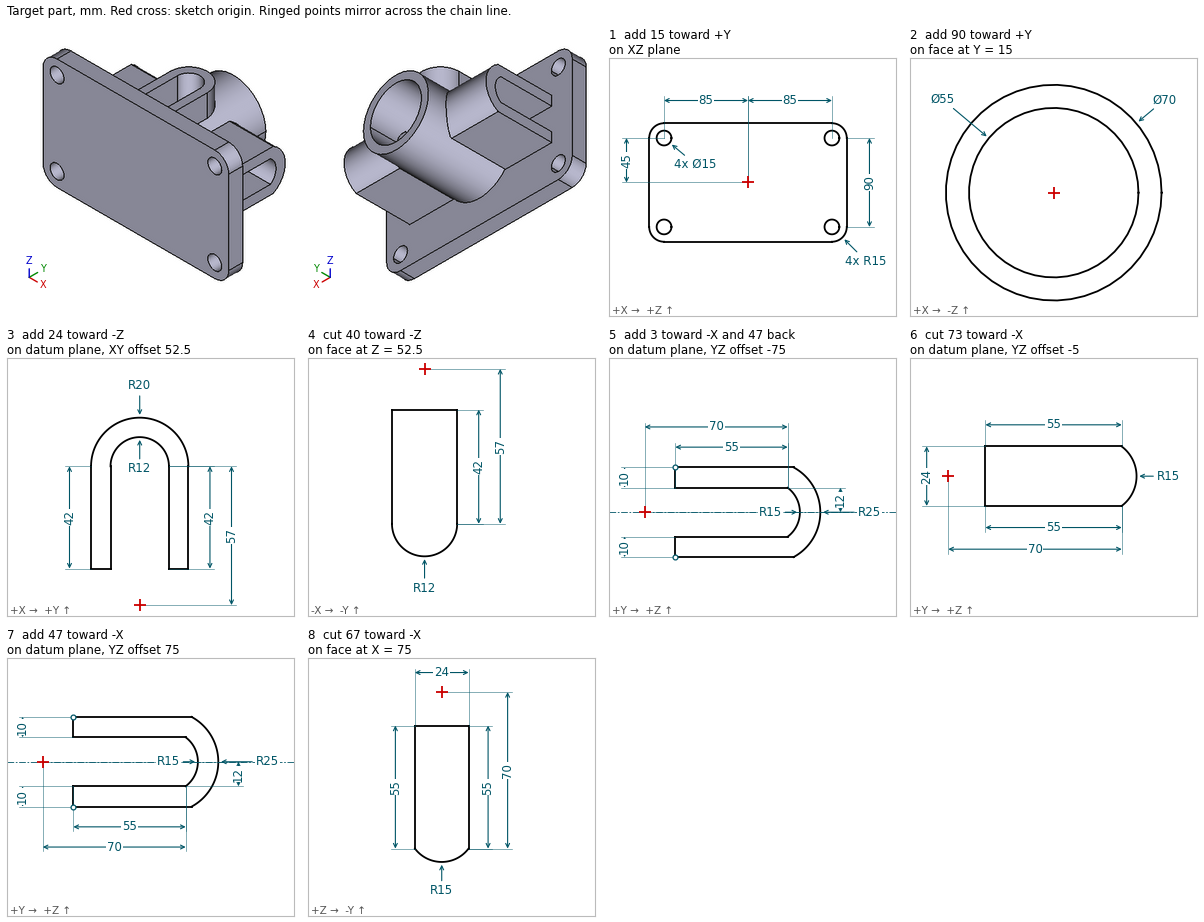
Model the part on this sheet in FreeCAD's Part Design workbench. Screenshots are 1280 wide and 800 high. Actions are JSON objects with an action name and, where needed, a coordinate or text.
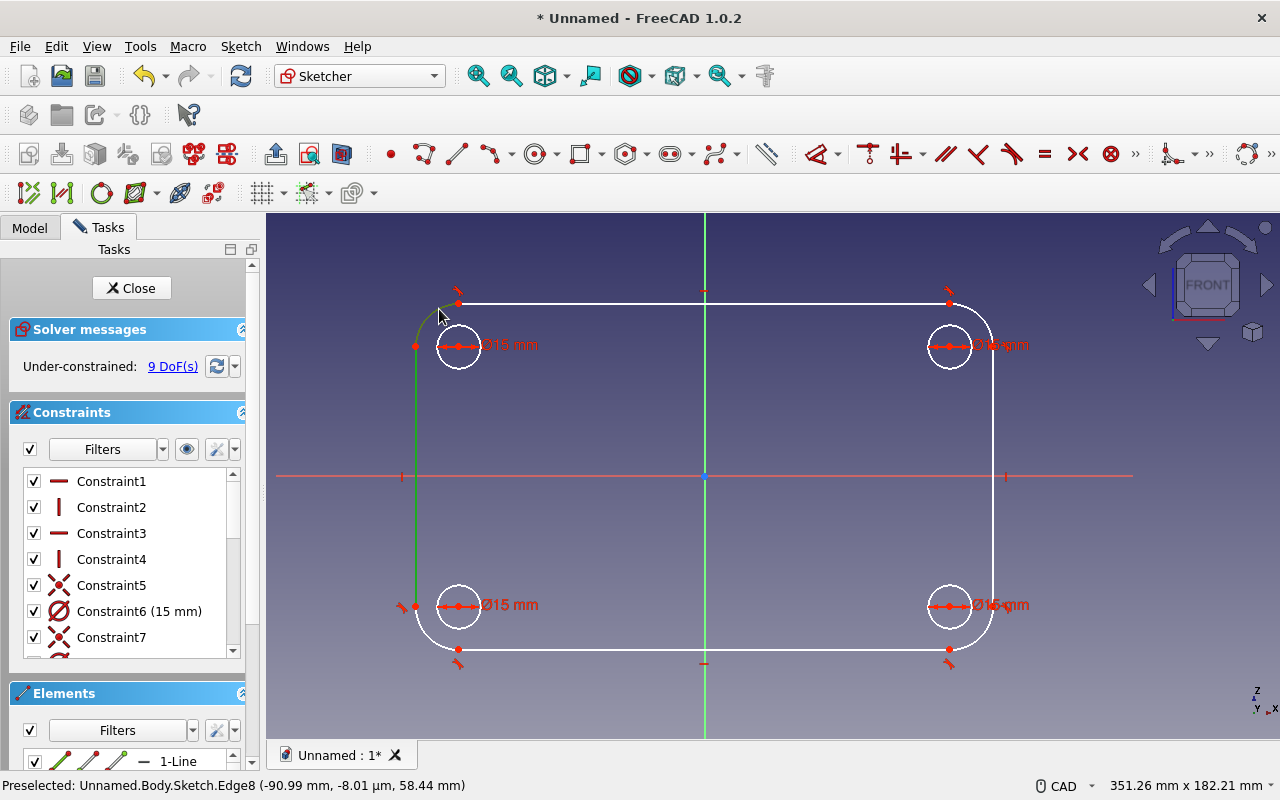
{"action": "key", "text": "t"}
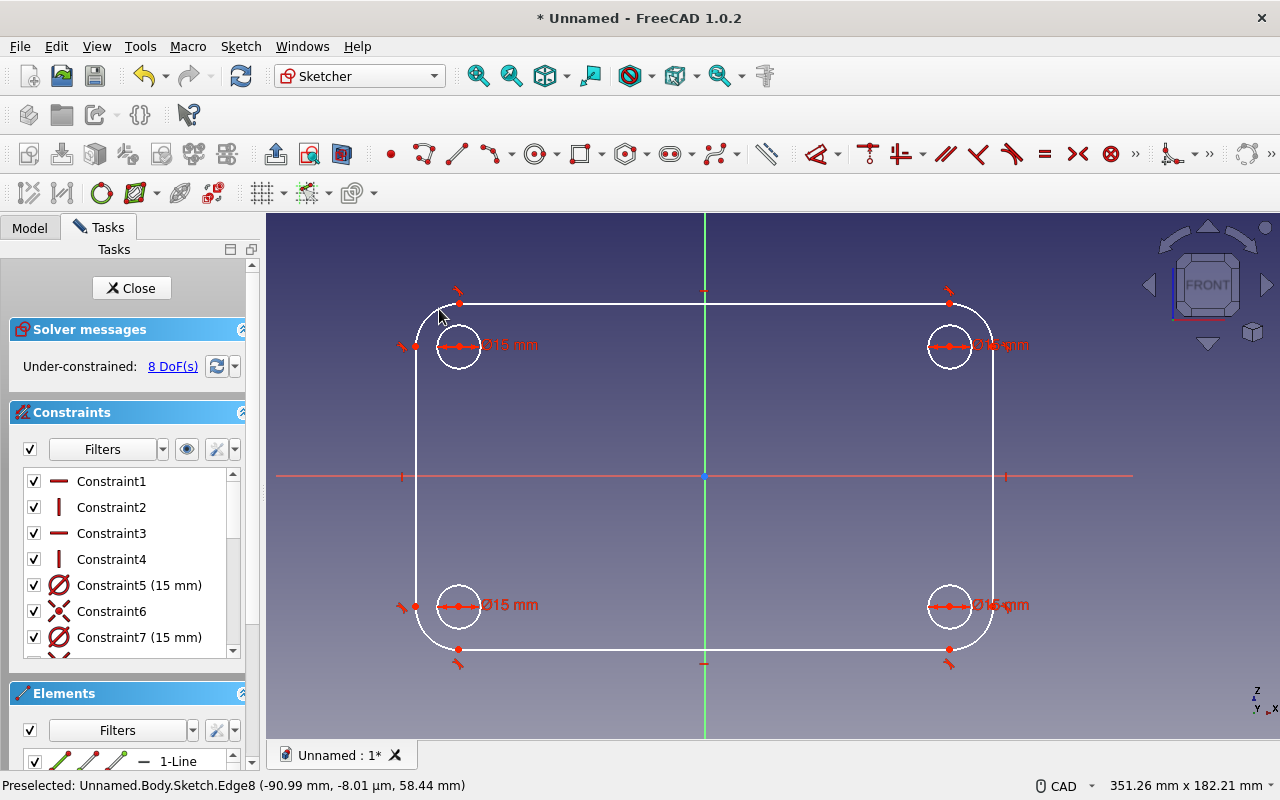
{"action": "left_click", "coordinate": [988, 327]}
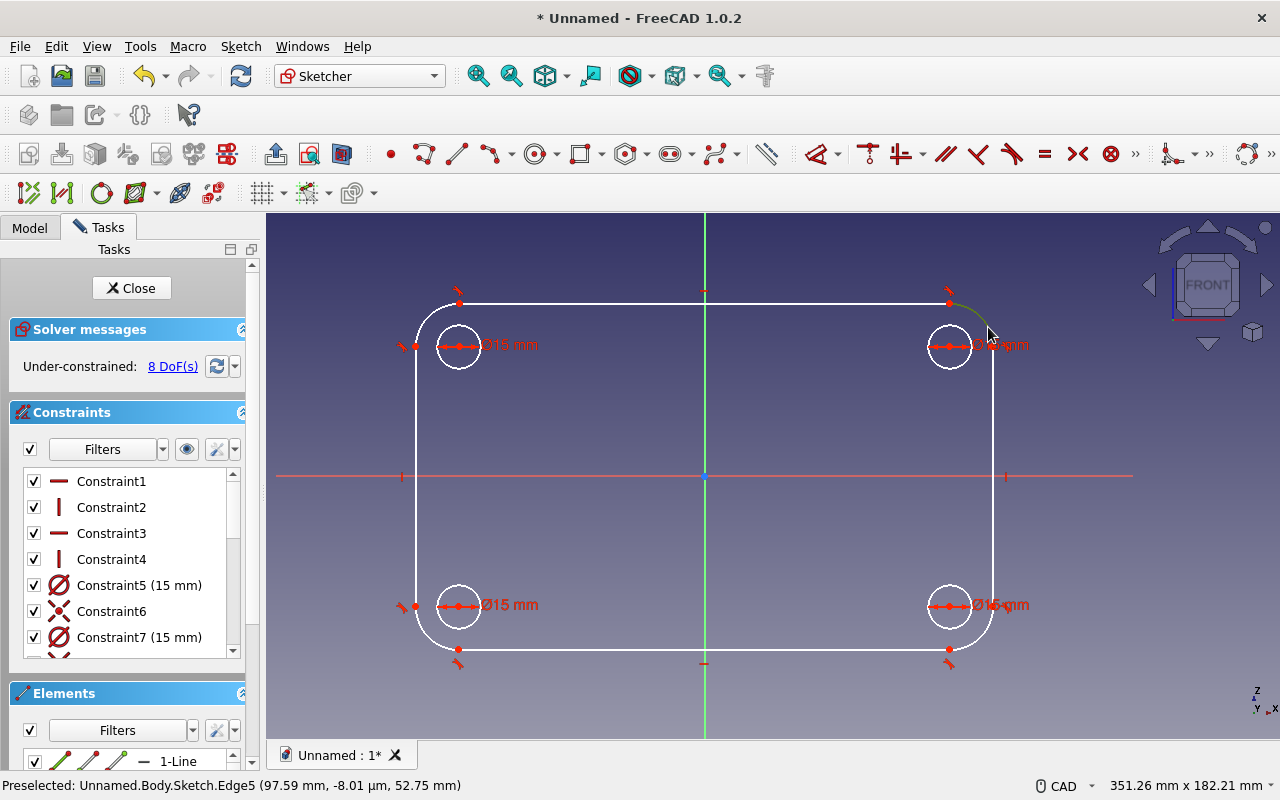
{"action": "left_click", "coordinate": [970, 645]}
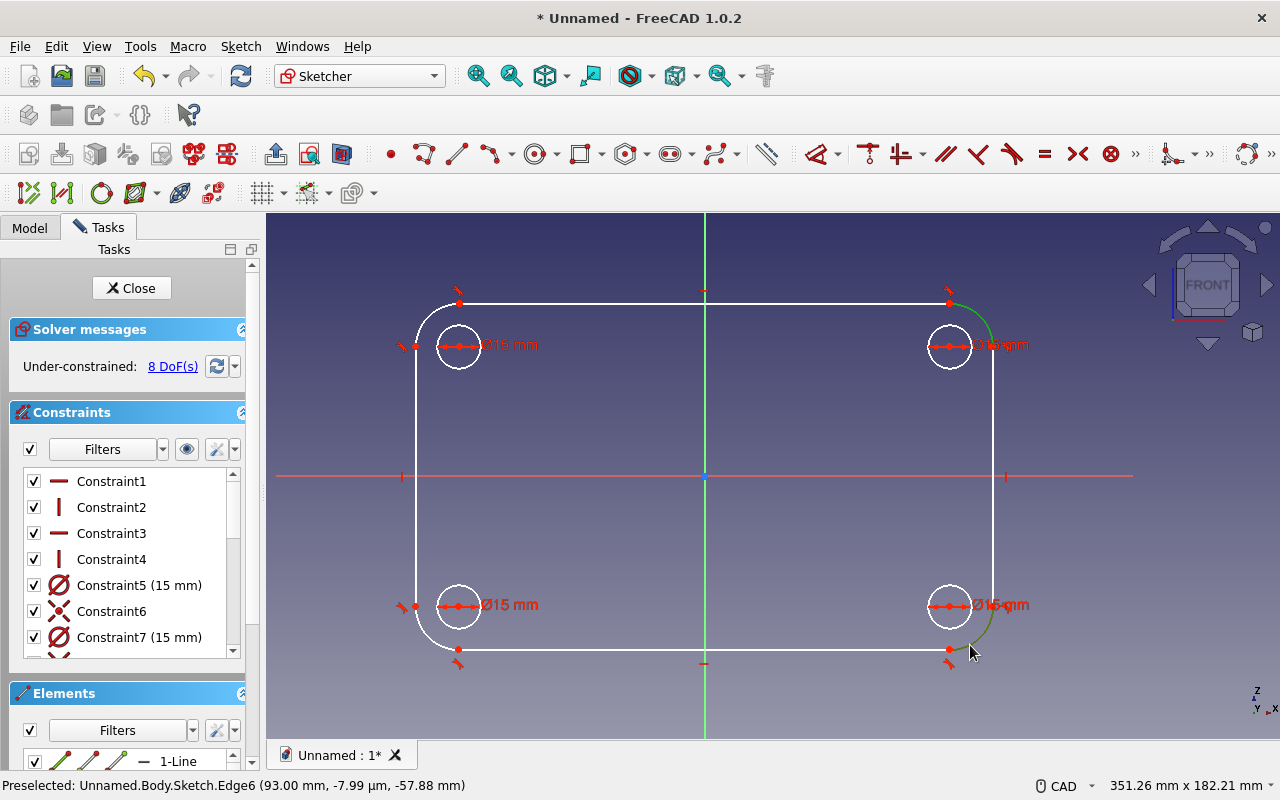
{"action": "left_click", "coordinate": [421, 627]}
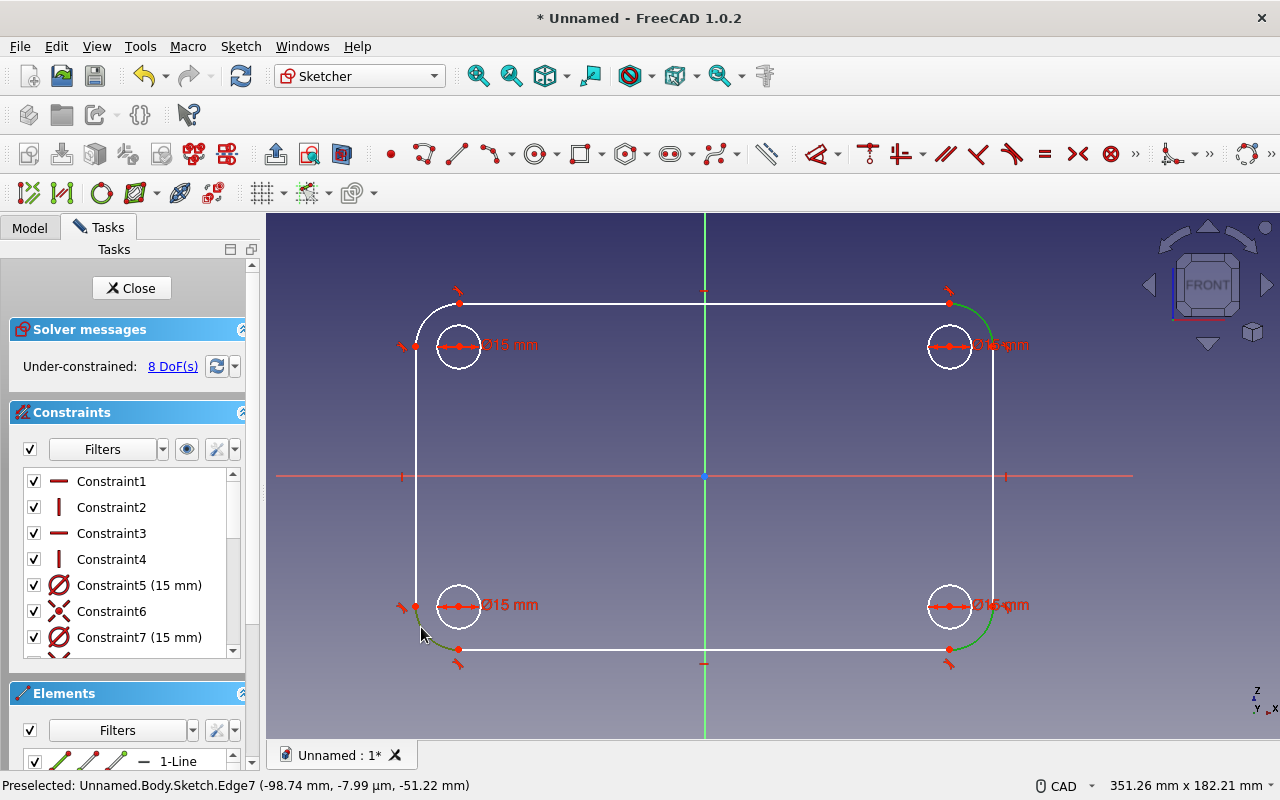
{"action": "left_click", "coordinate": [439, 309]}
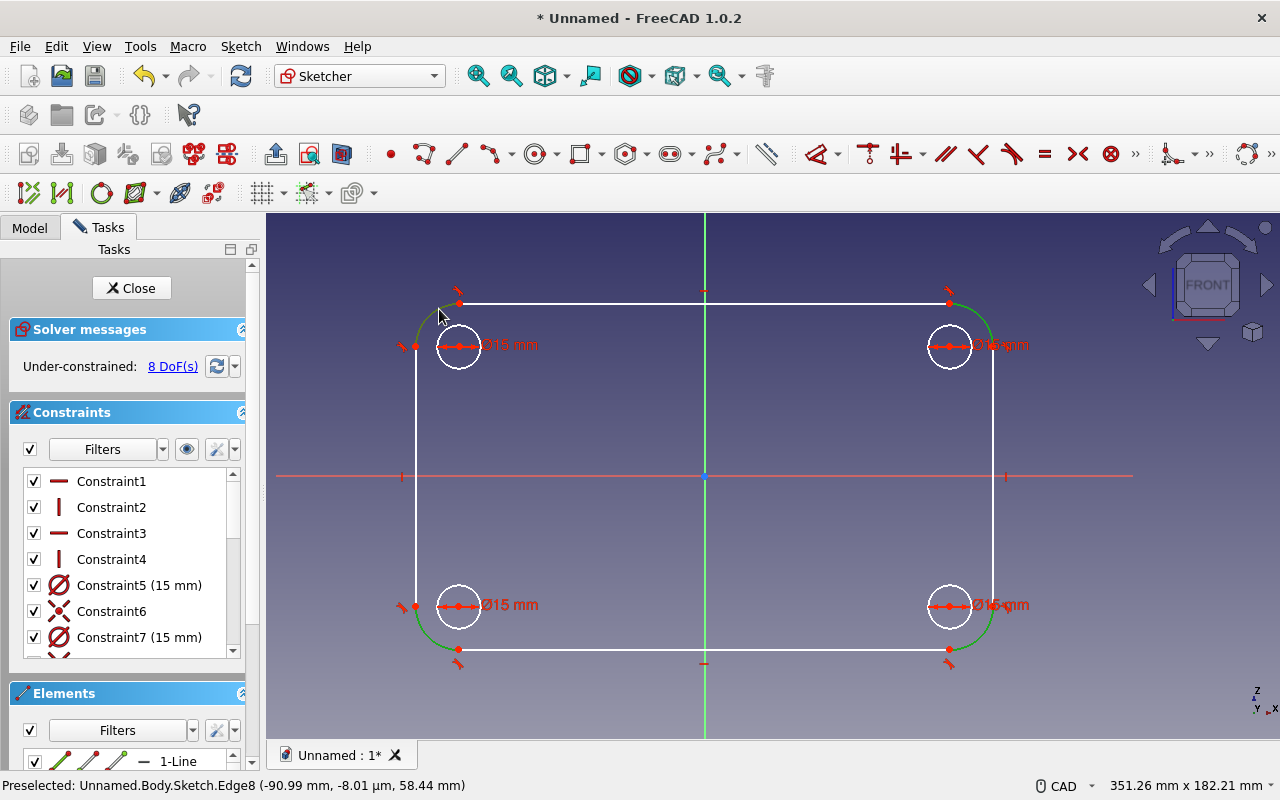
{"action": "key", "text": "e"}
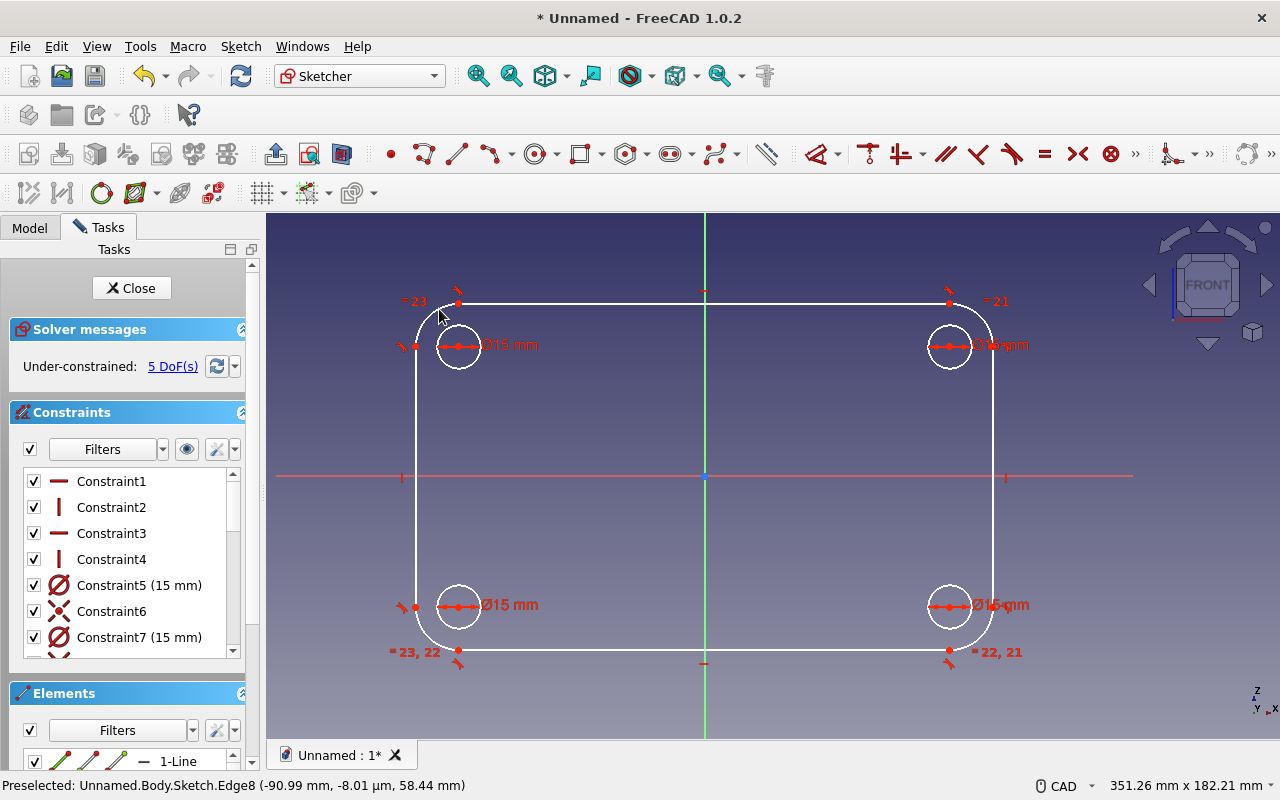
{"action": "left_click", "coordinate": [988, 327]}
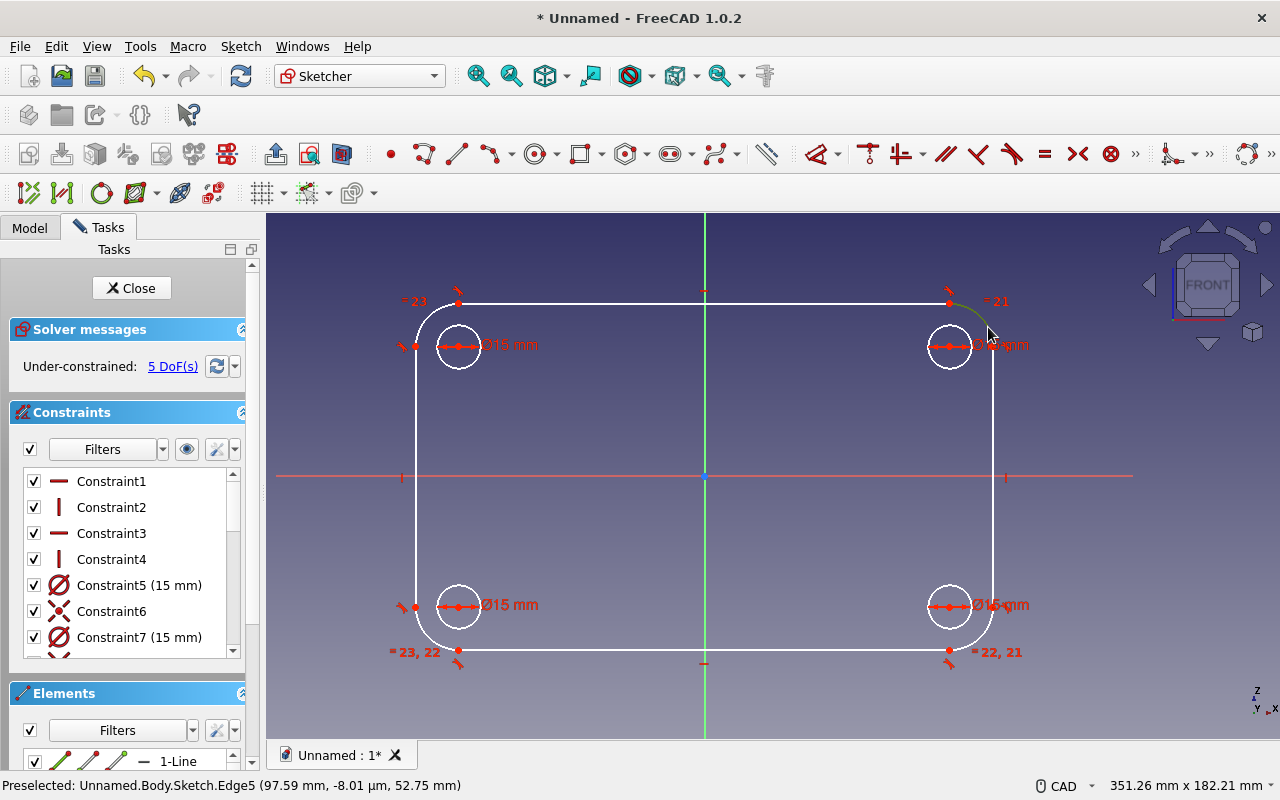
{"action": "key", "text": "k r"}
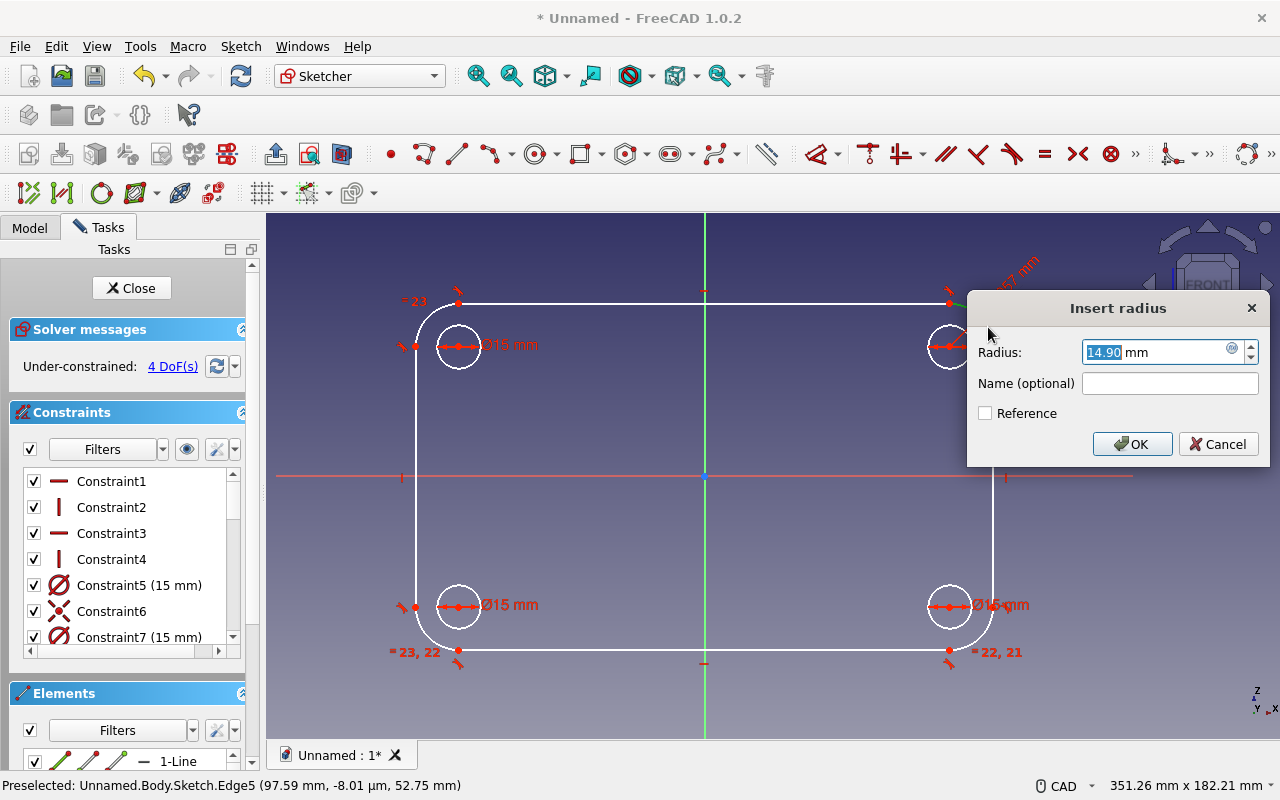
{"action": "type", "text": "15"}
{"action": "key", "text": "Return"}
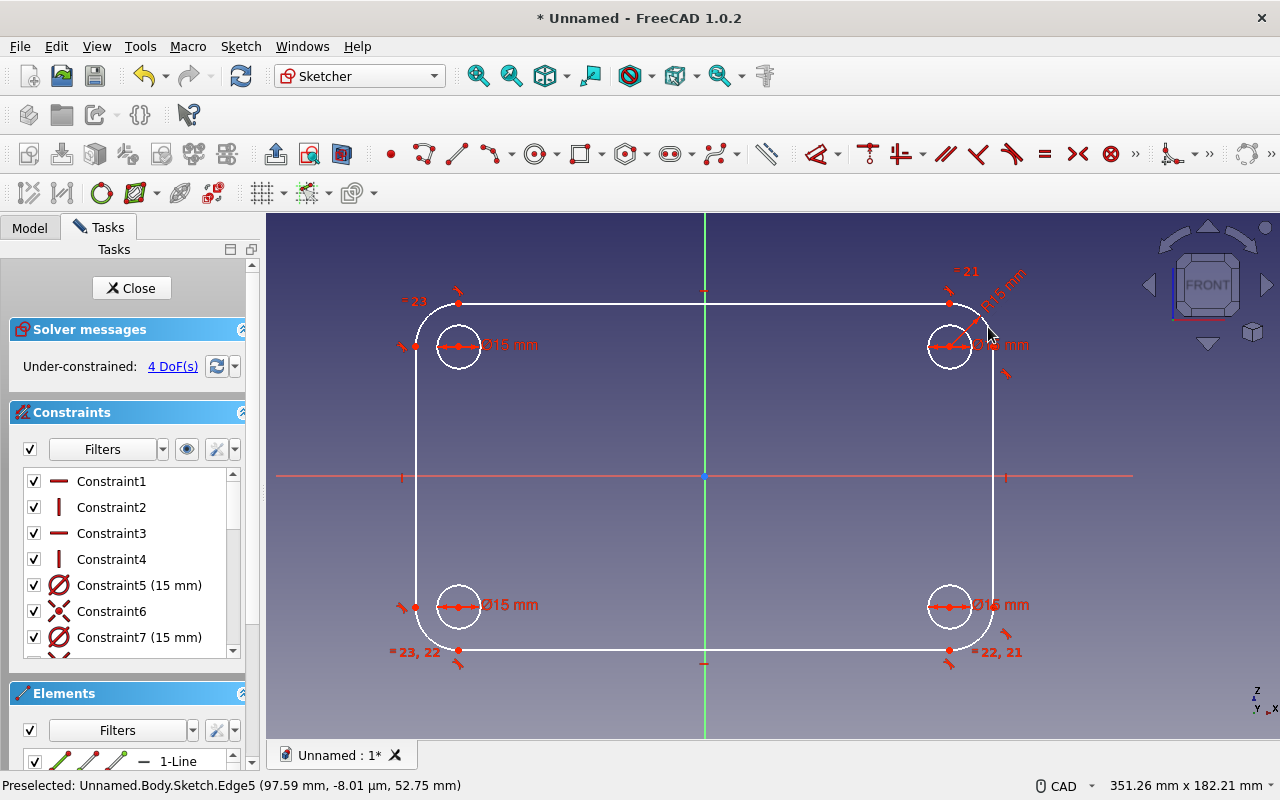
{"action": "left_click", "coordinate": [993, 425]}